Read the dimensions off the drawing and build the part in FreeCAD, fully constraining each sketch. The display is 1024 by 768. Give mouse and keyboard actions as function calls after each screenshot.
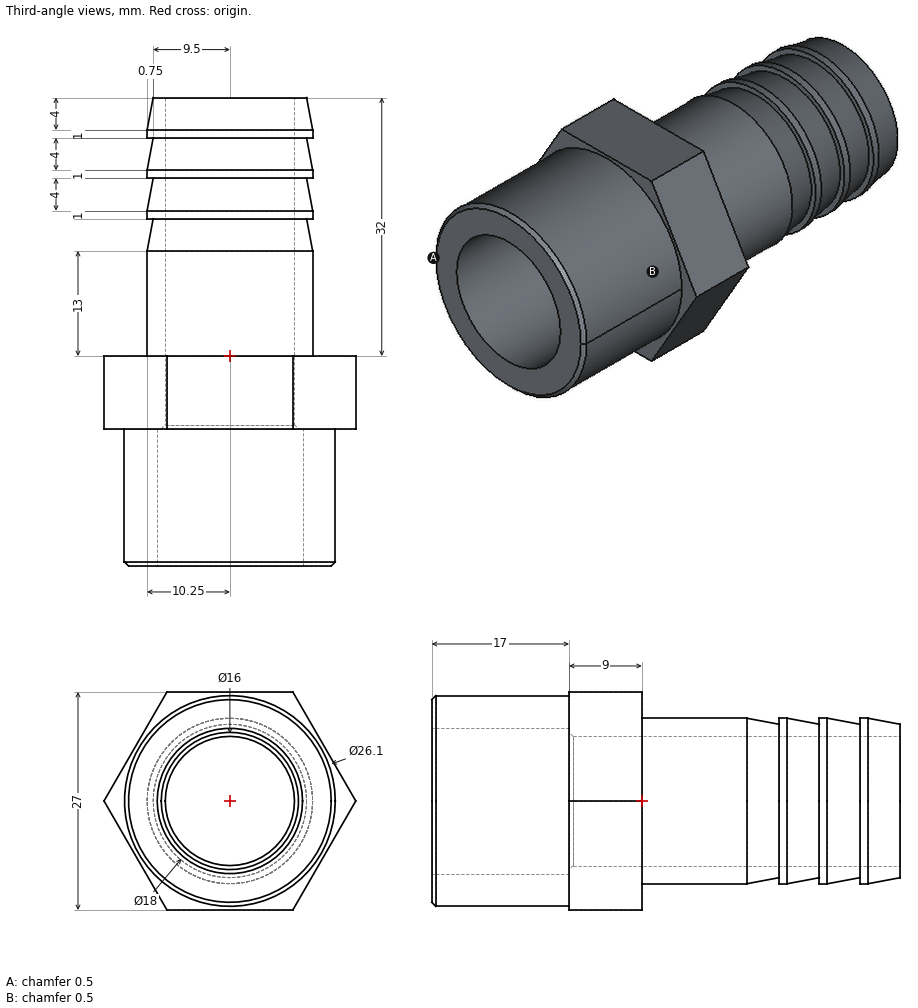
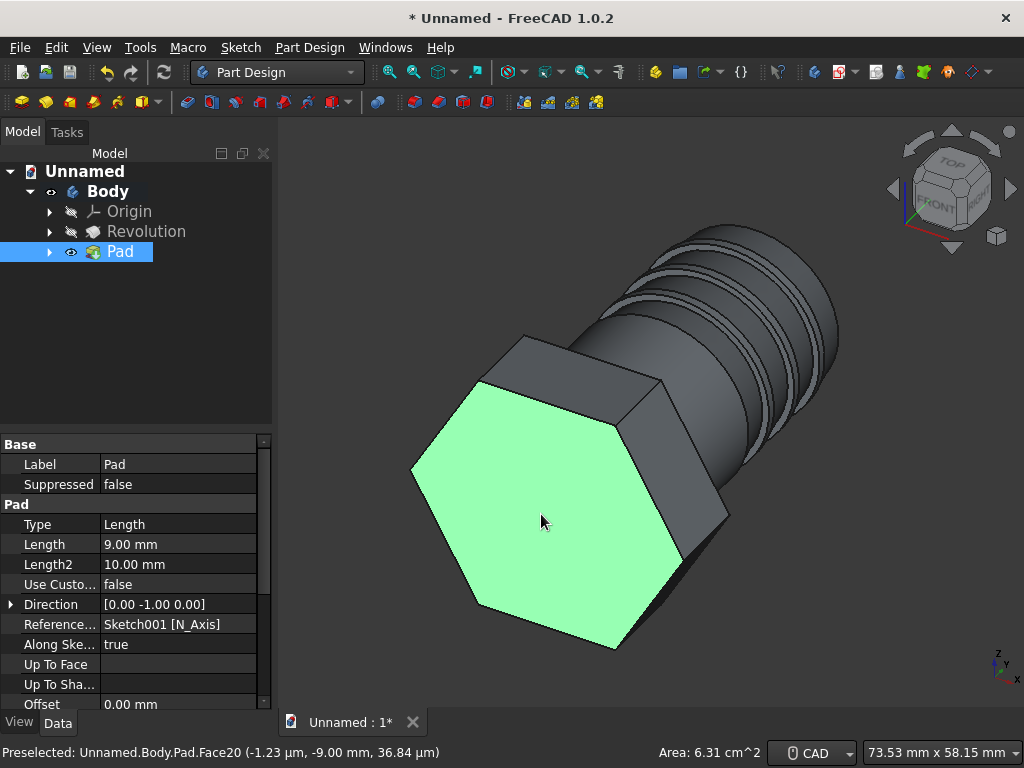
click(840, 72)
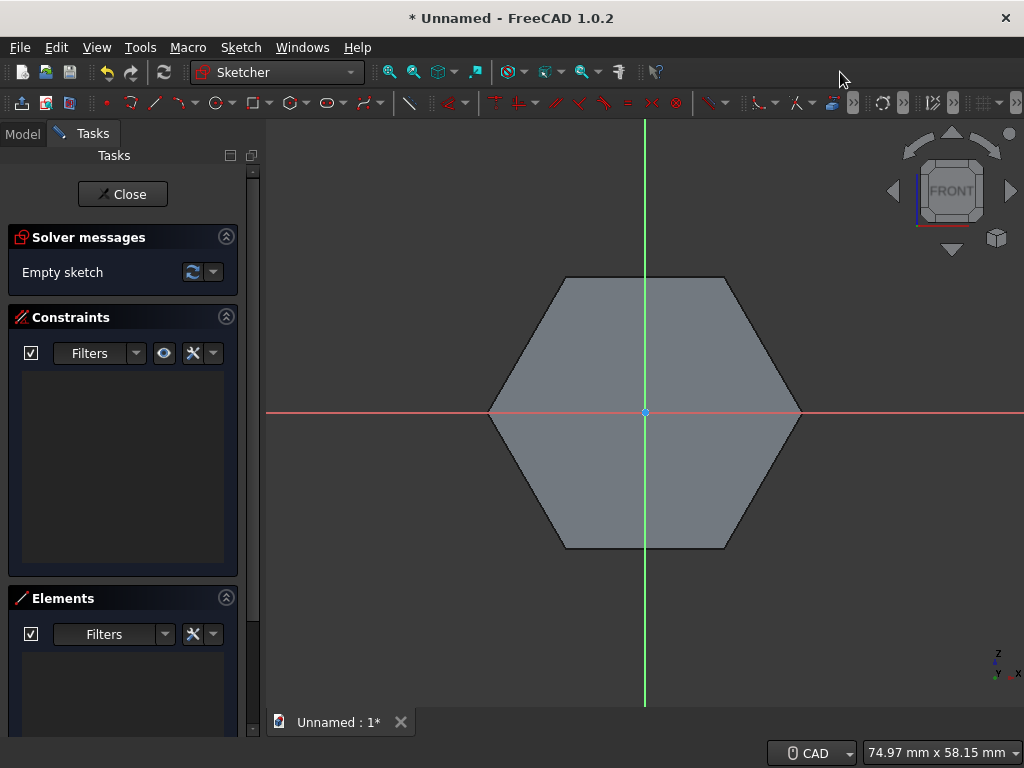
scroll(784, 413, up, 2)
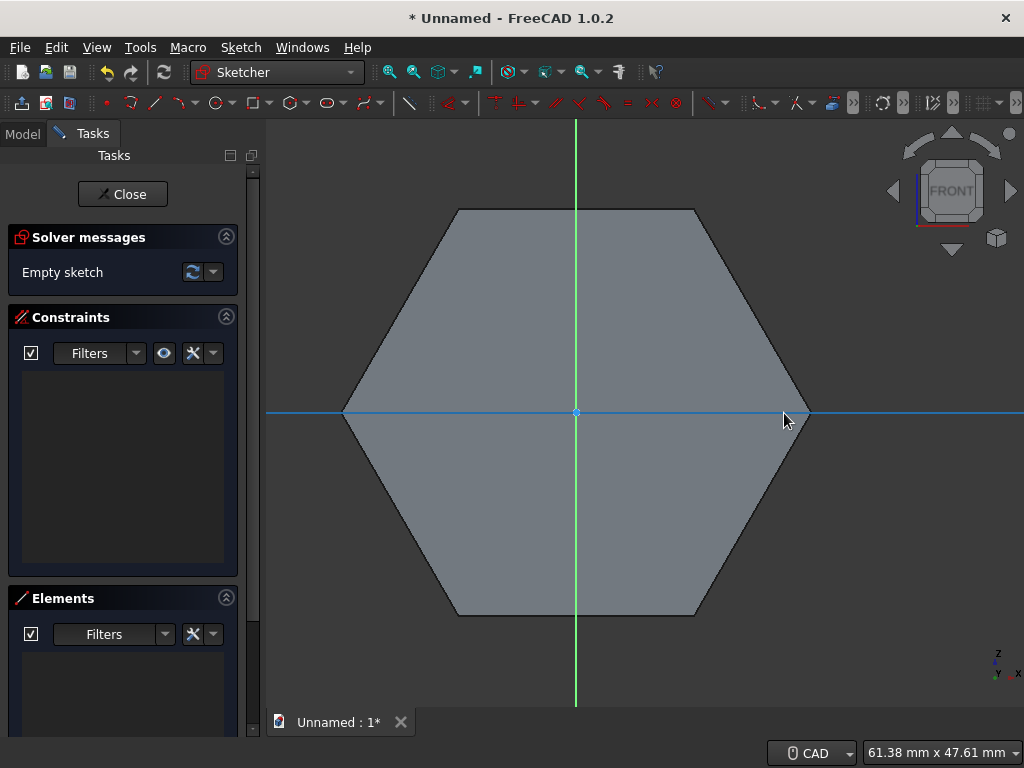
key(g)
key(c)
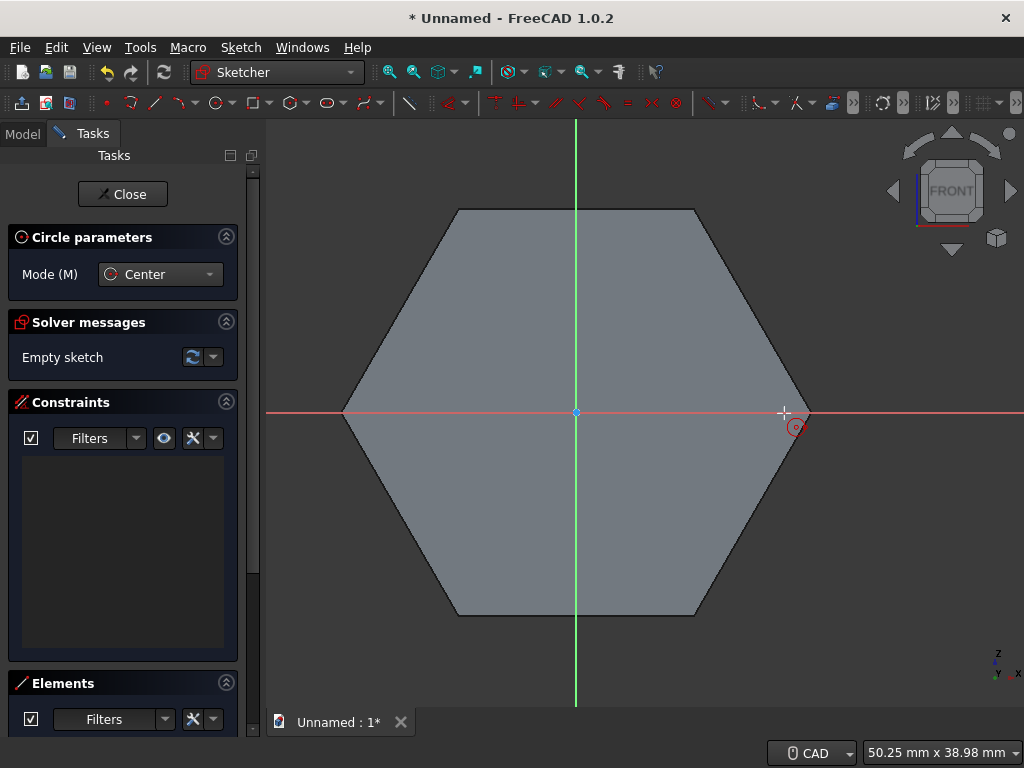
click(576, 413)
click(715, 274)
key(Escape)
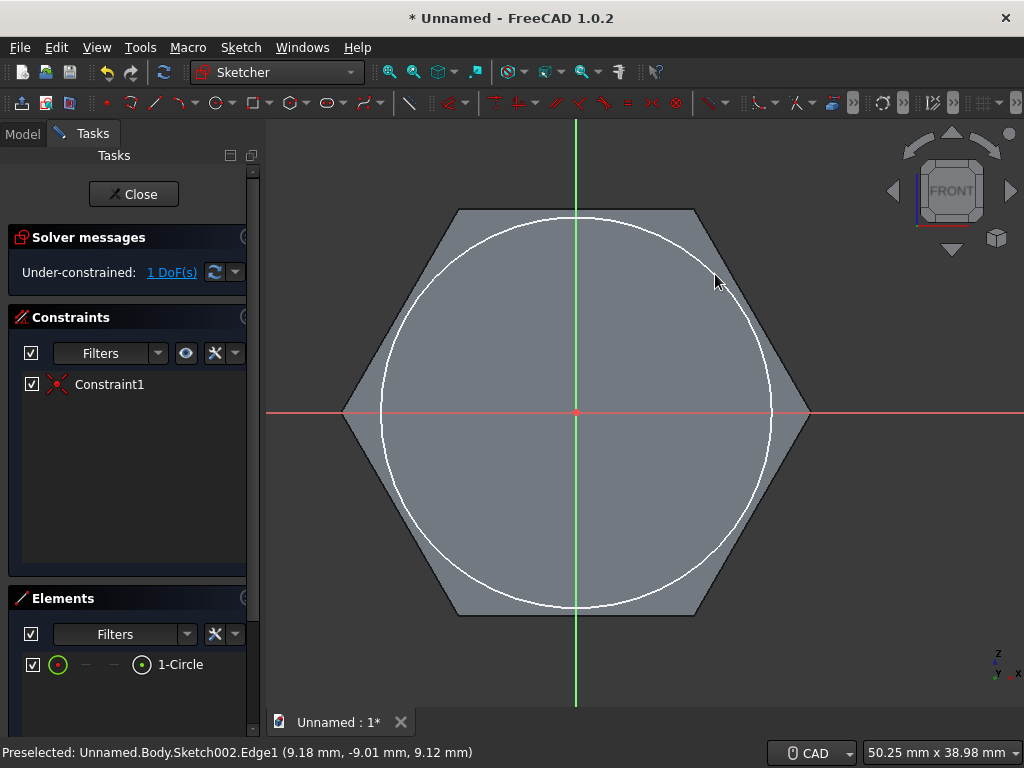
key(d)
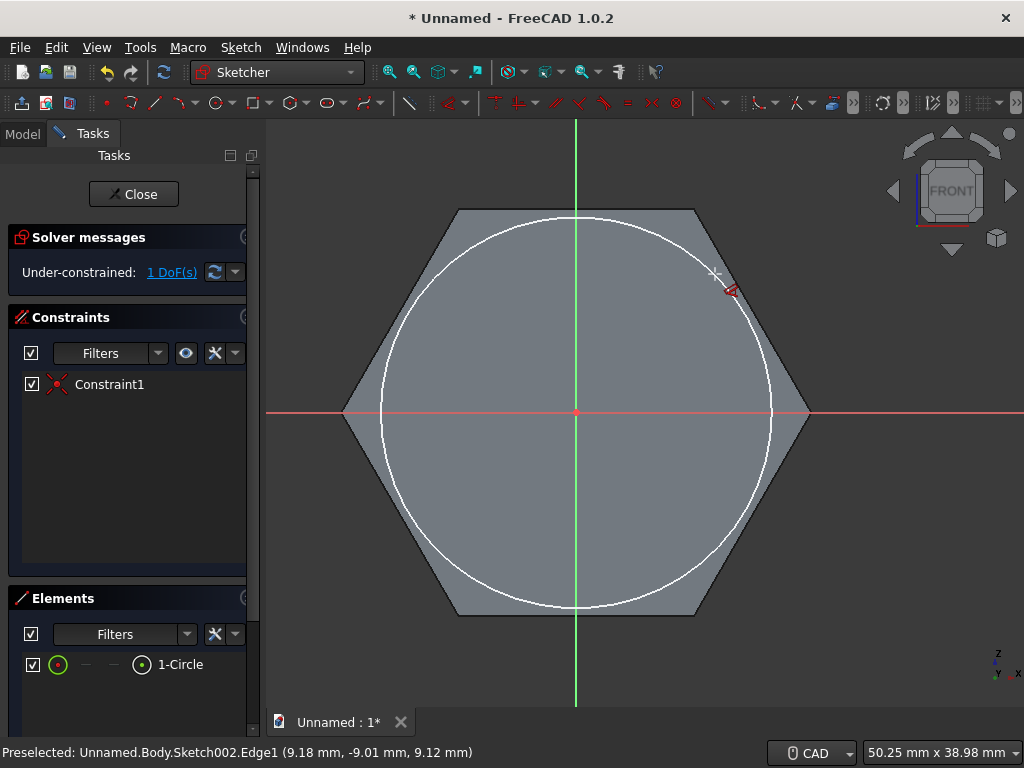
click(714, 274)
click(737, 251)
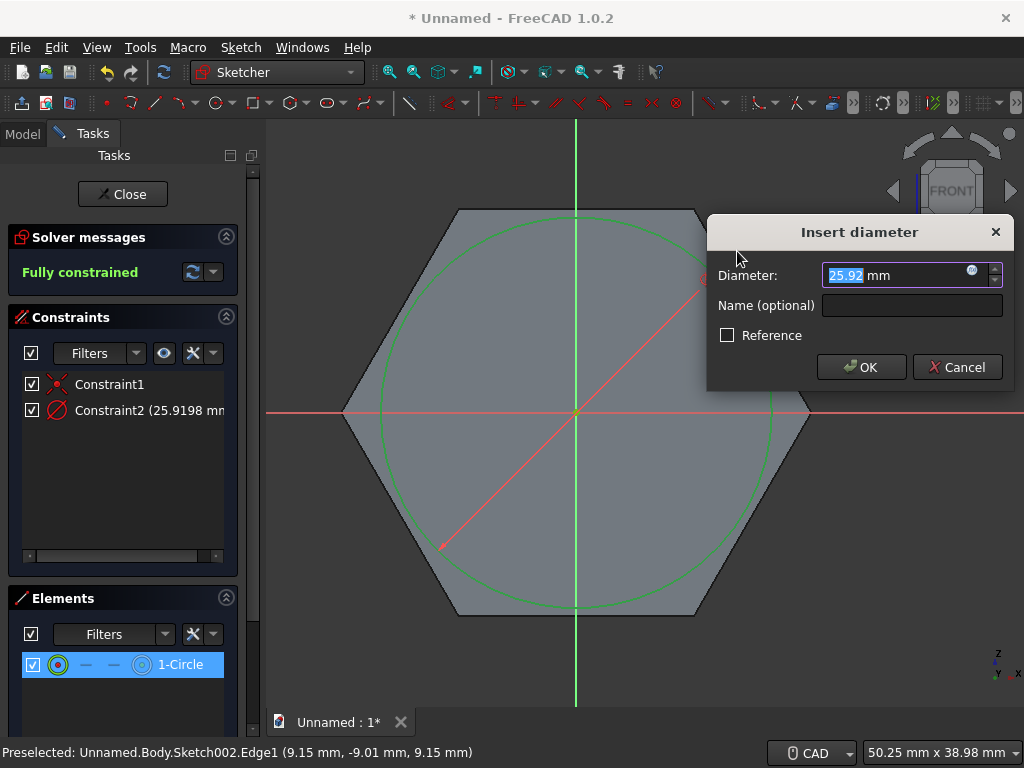
text(26.1)
key(Return)
key(Escape)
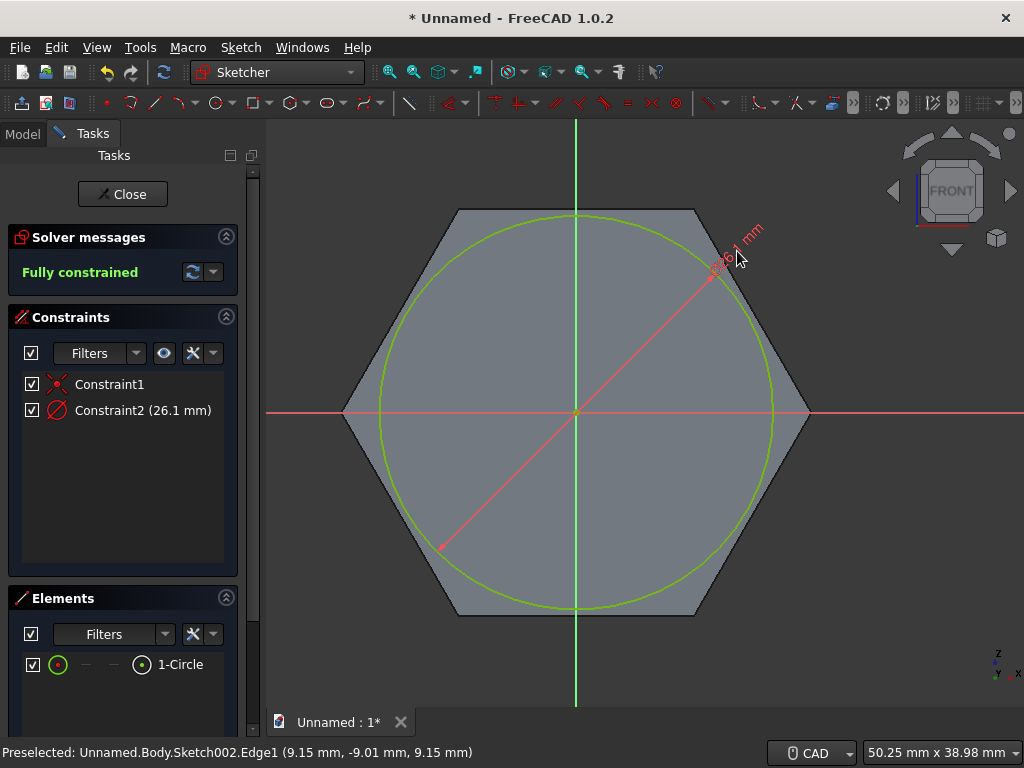
click(123, 194)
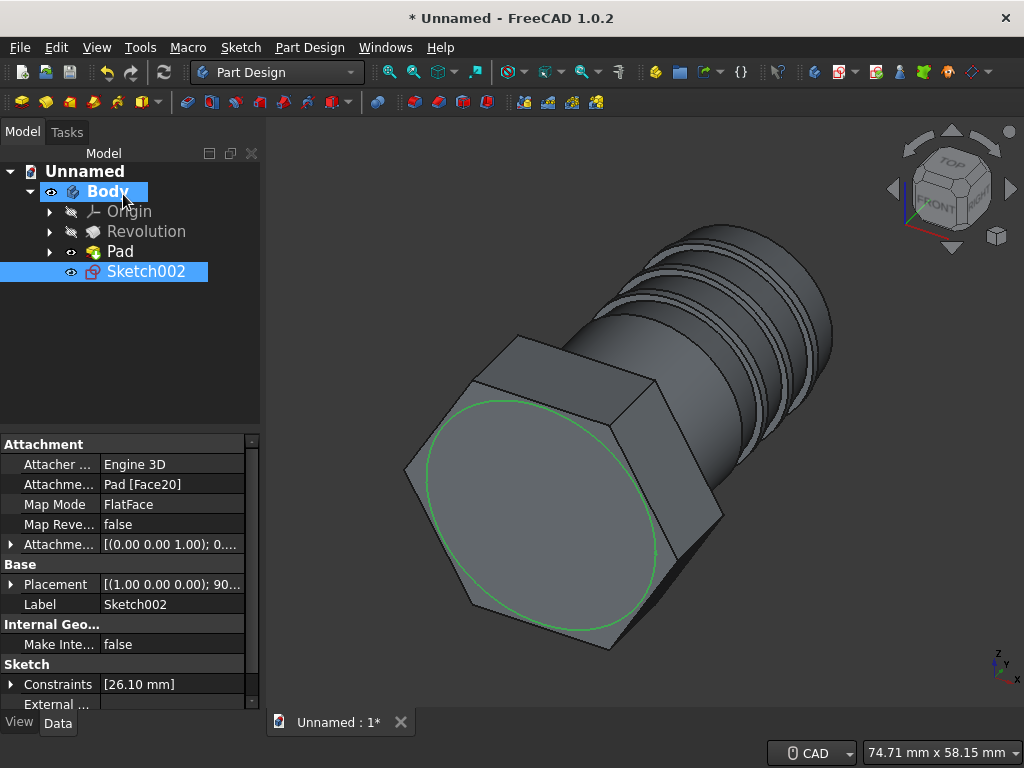
click(22, 102)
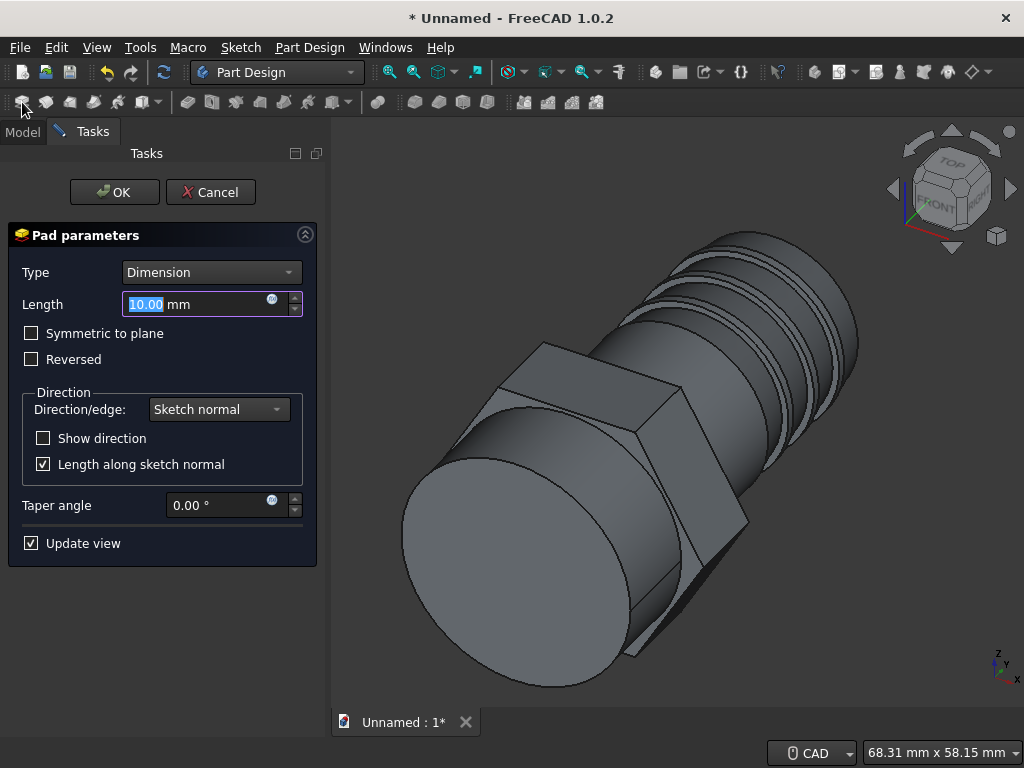
text(17)
key(Tab)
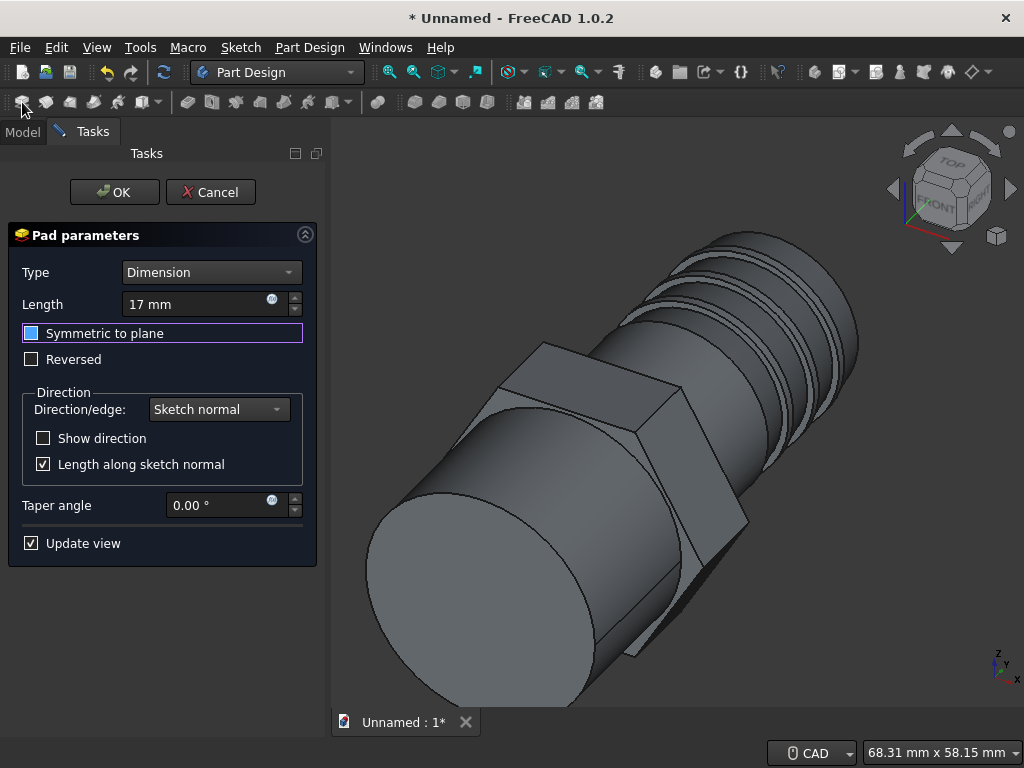
click(115, 192)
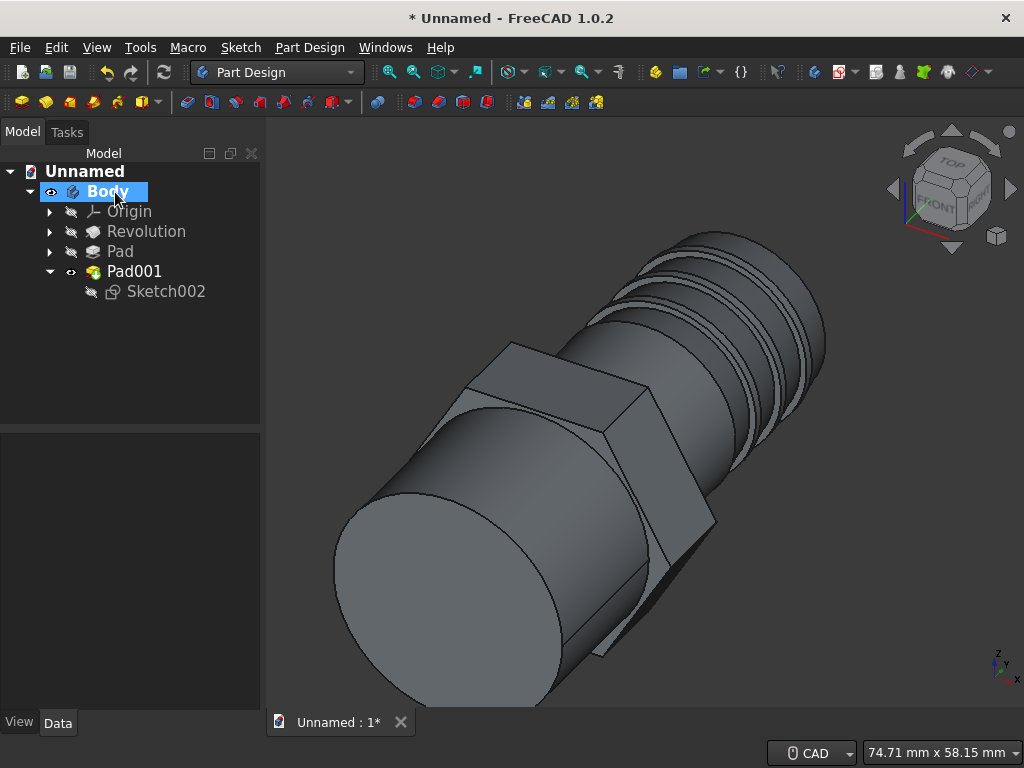
key(v)
key(f)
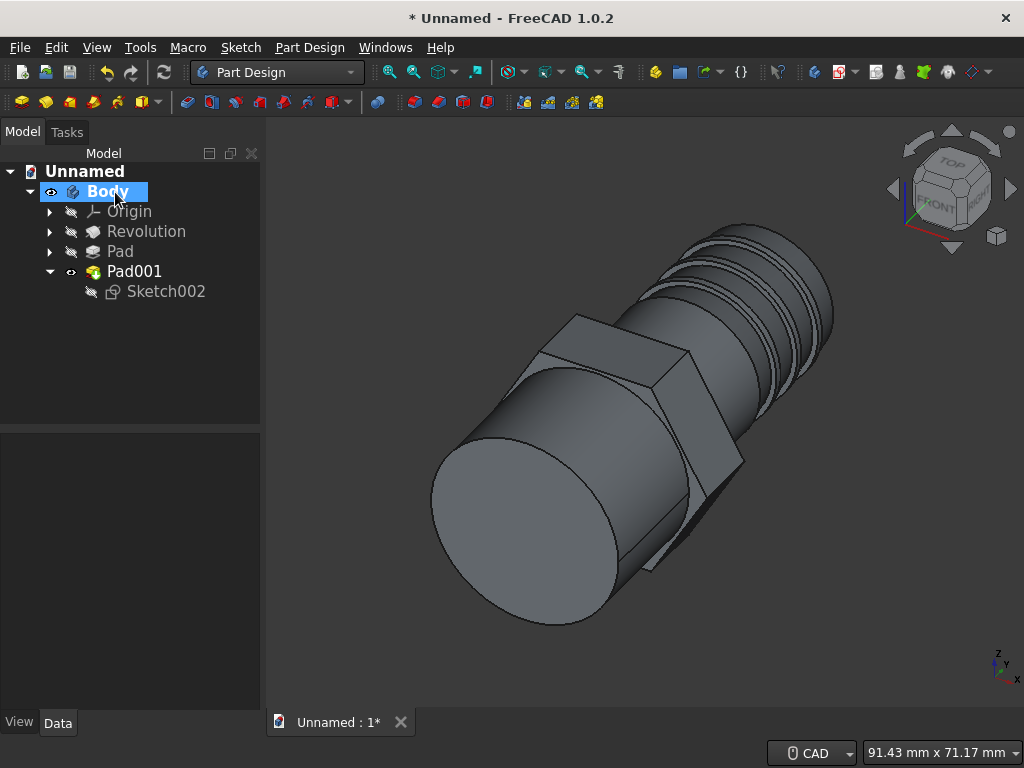
key(4)